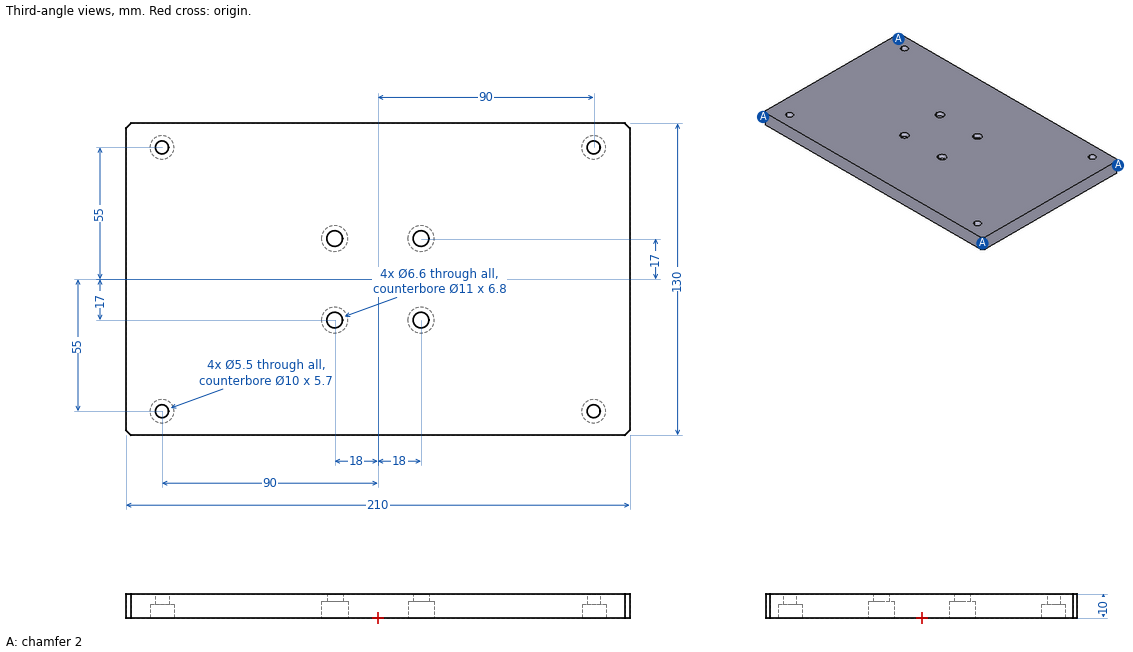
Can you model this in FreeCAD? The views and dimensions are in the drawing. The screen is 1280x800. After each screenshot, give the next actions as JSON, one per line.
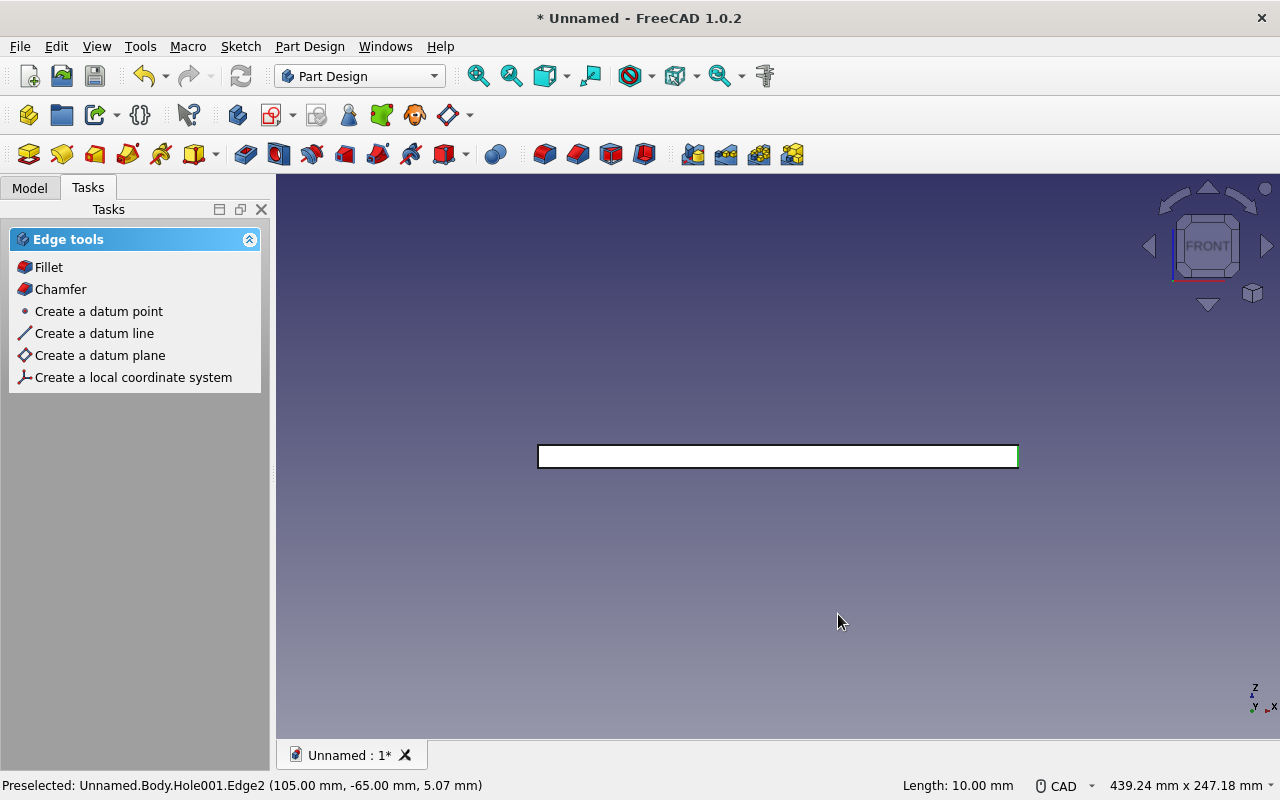
{"action": "left_click", "coordinate": [538, 455], "text": "ctrl"}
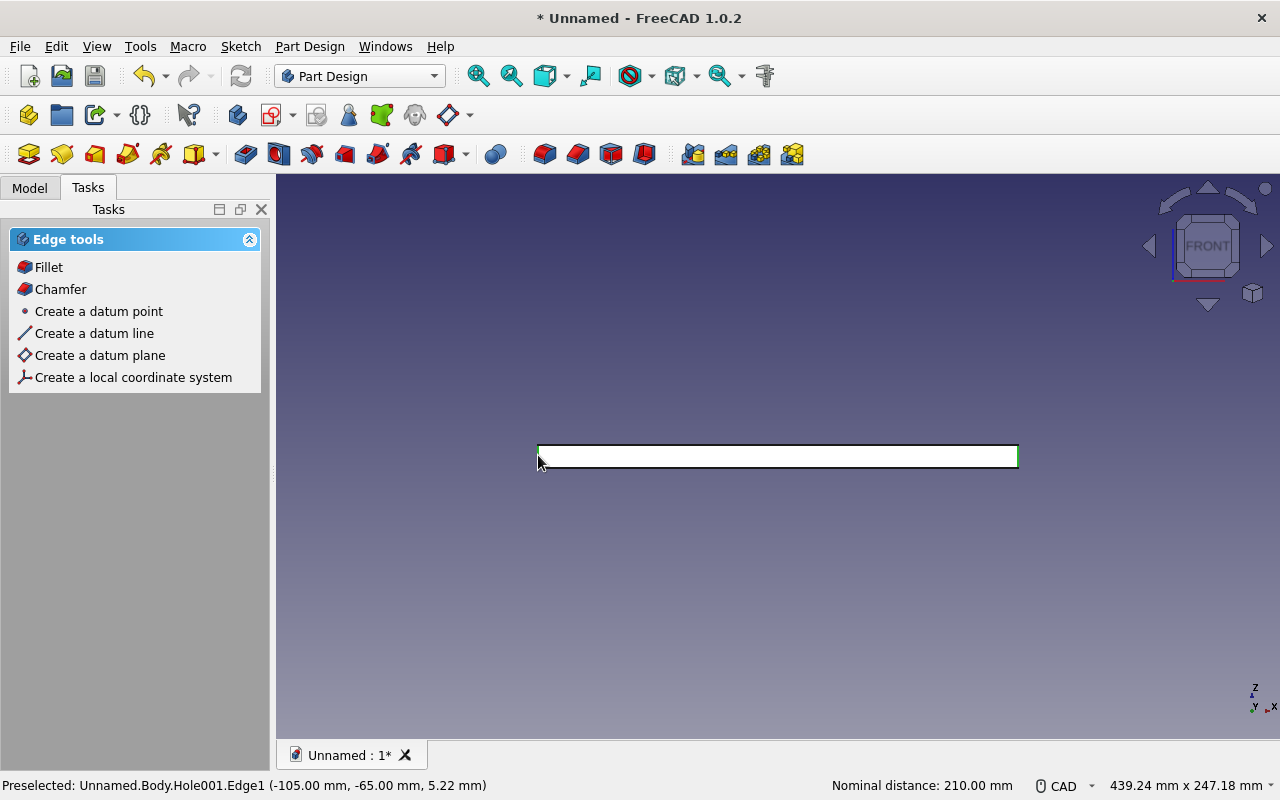
{"action": "key", "text": "3"}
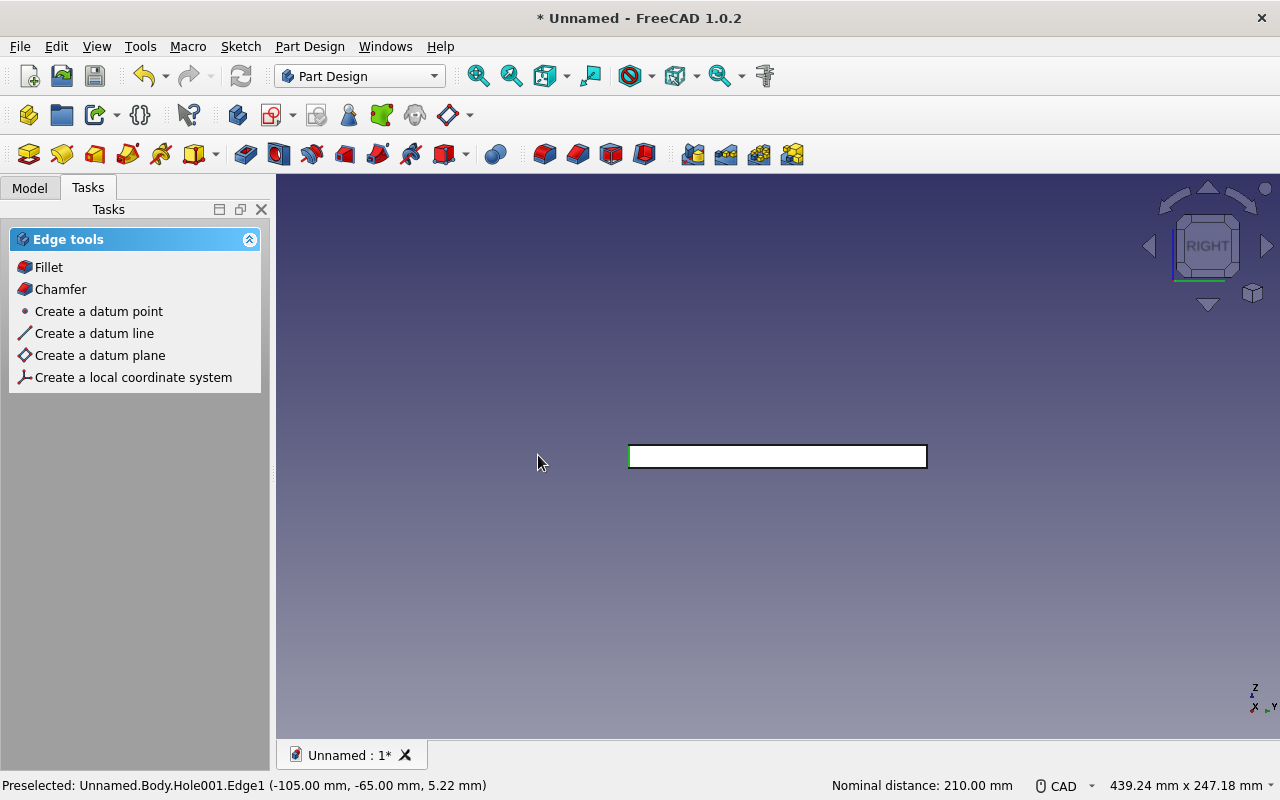
{"action": "left_click", "coordinate": [479, 76]}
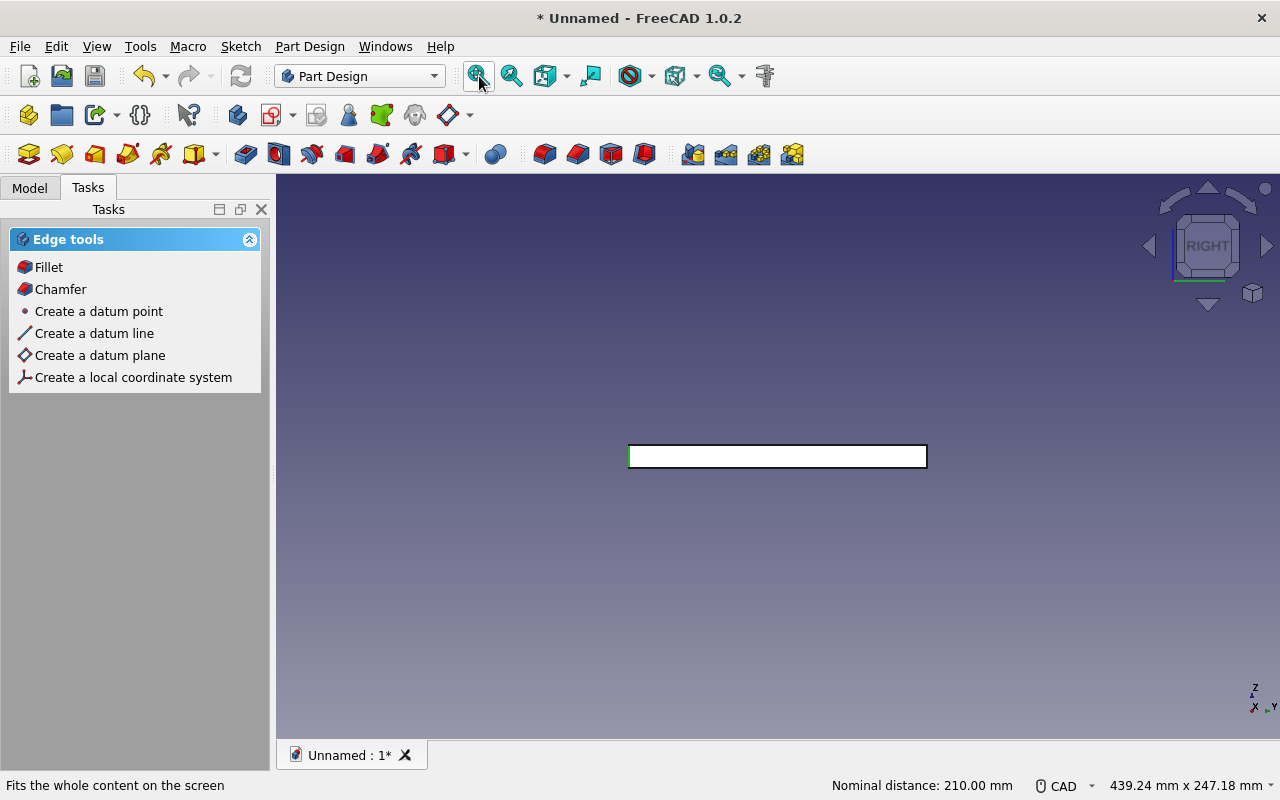
{"action": "left_click", "coordinate": [927, 455], "text": "ctrl"}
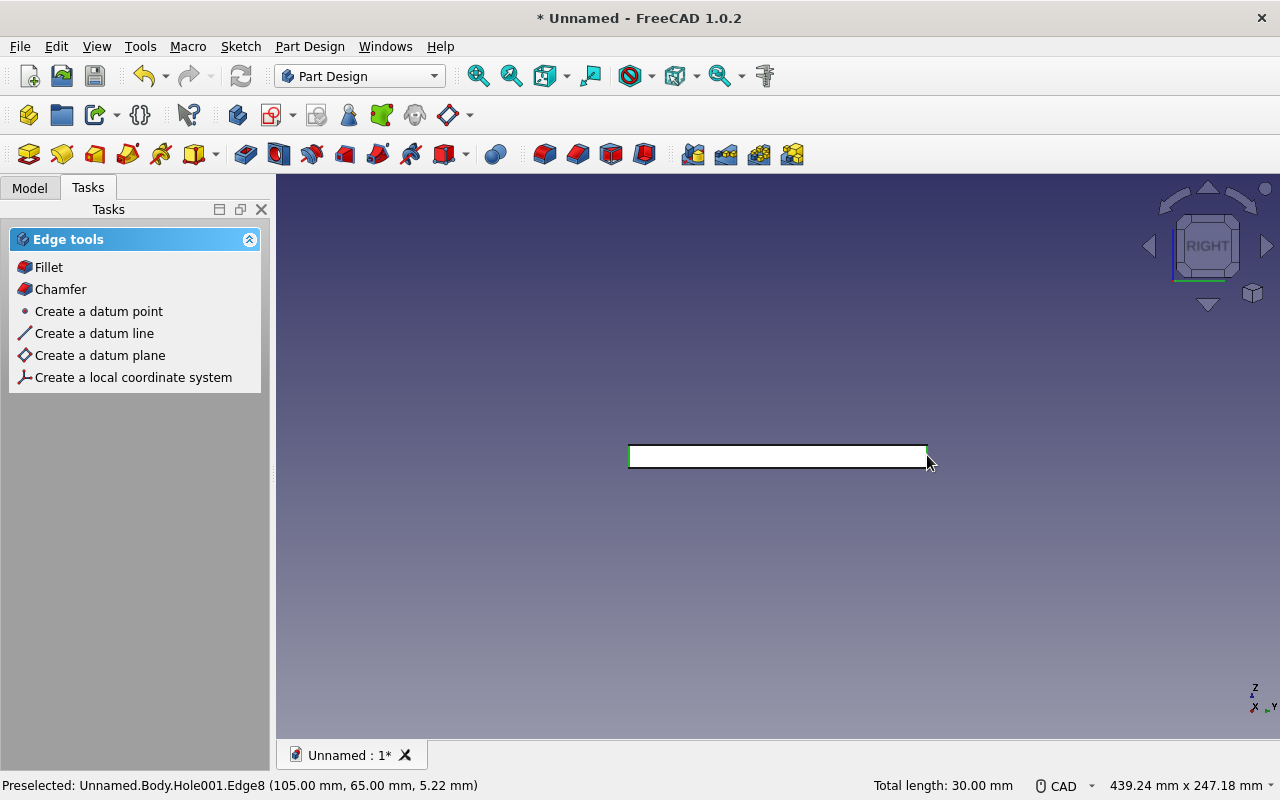
{"action": "key", "text": "5"}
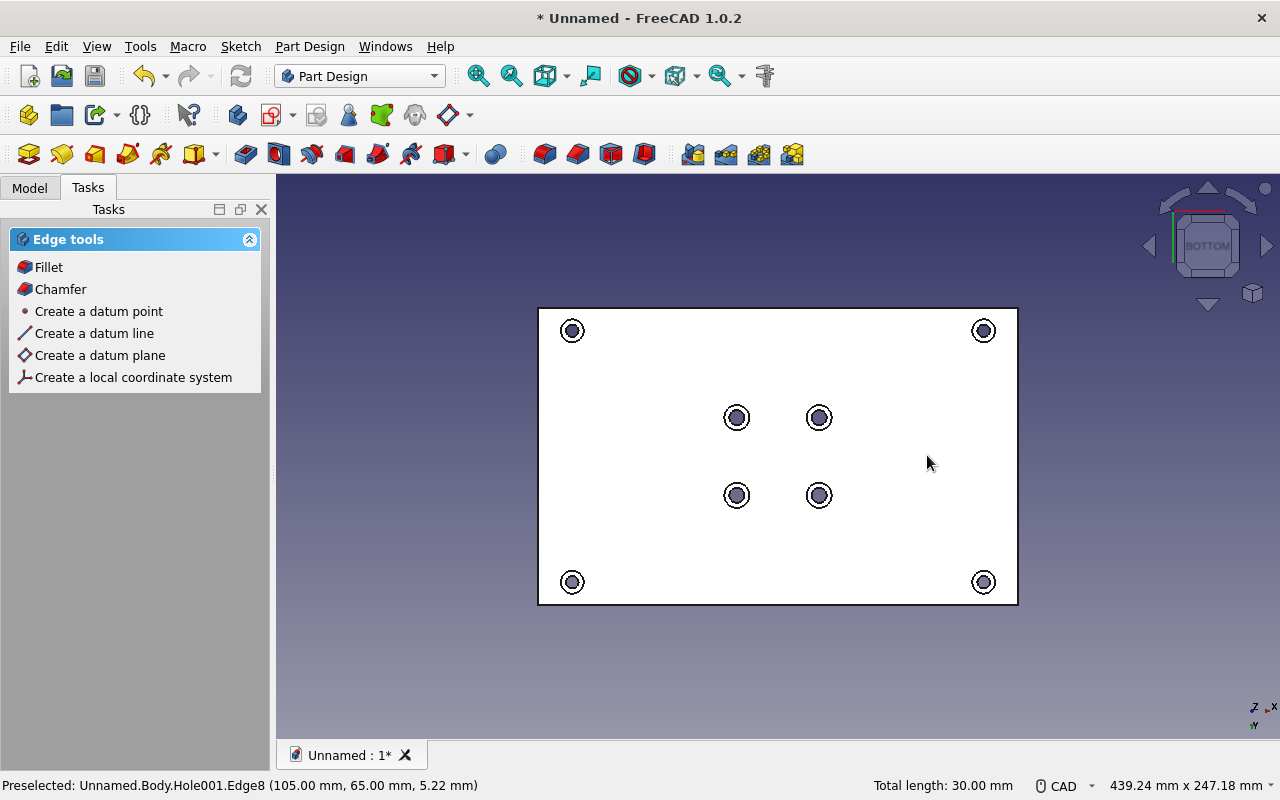
{"action": "key", "text": "4"}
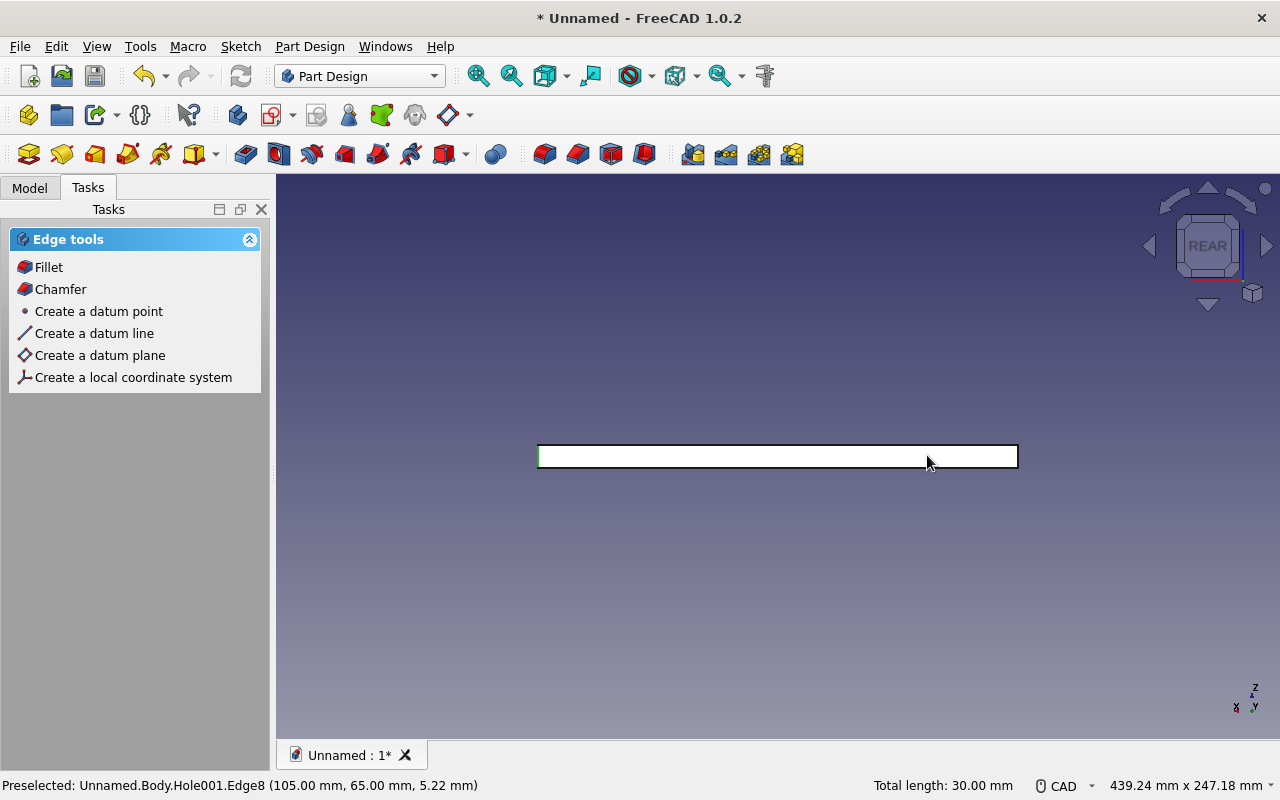
{"action": "left_click", "coordinate": [1018, 455], "text": "ctrl"}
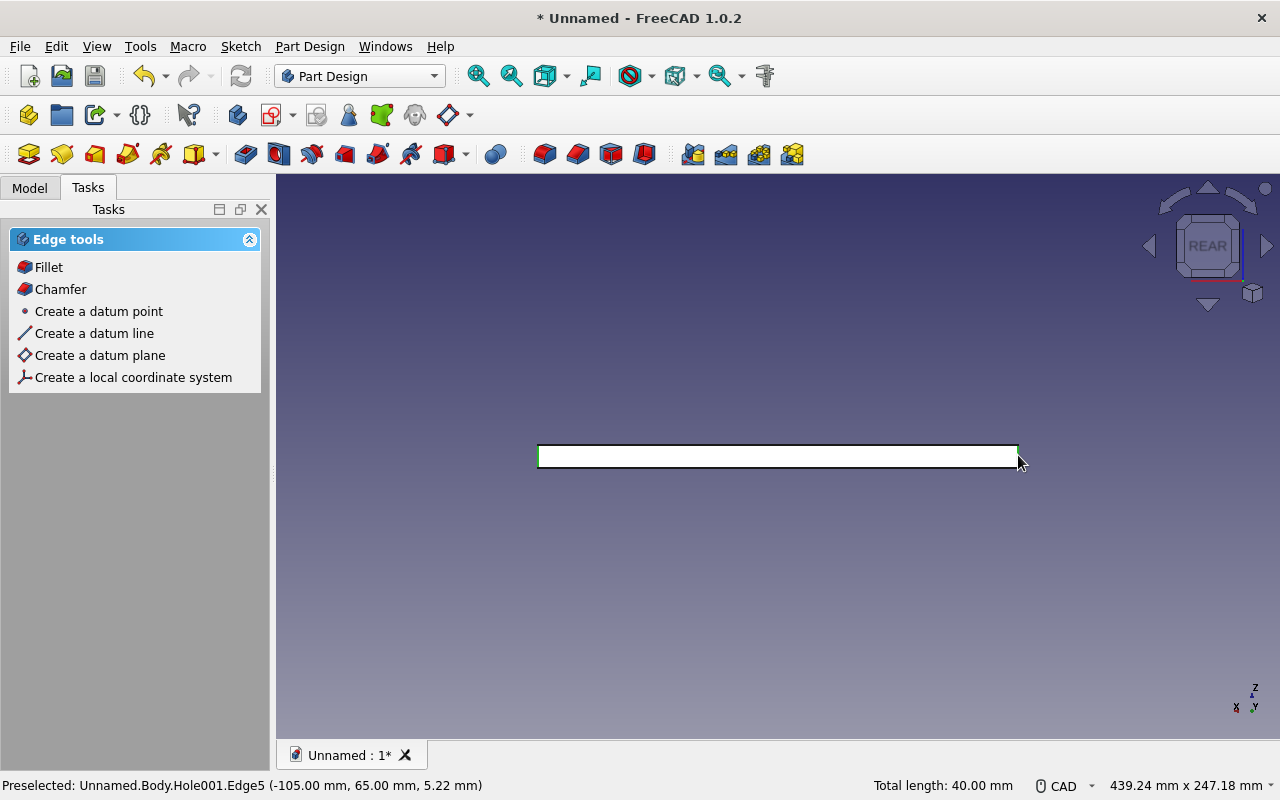
{"action": "left_click", "coordinate": [578, 154]}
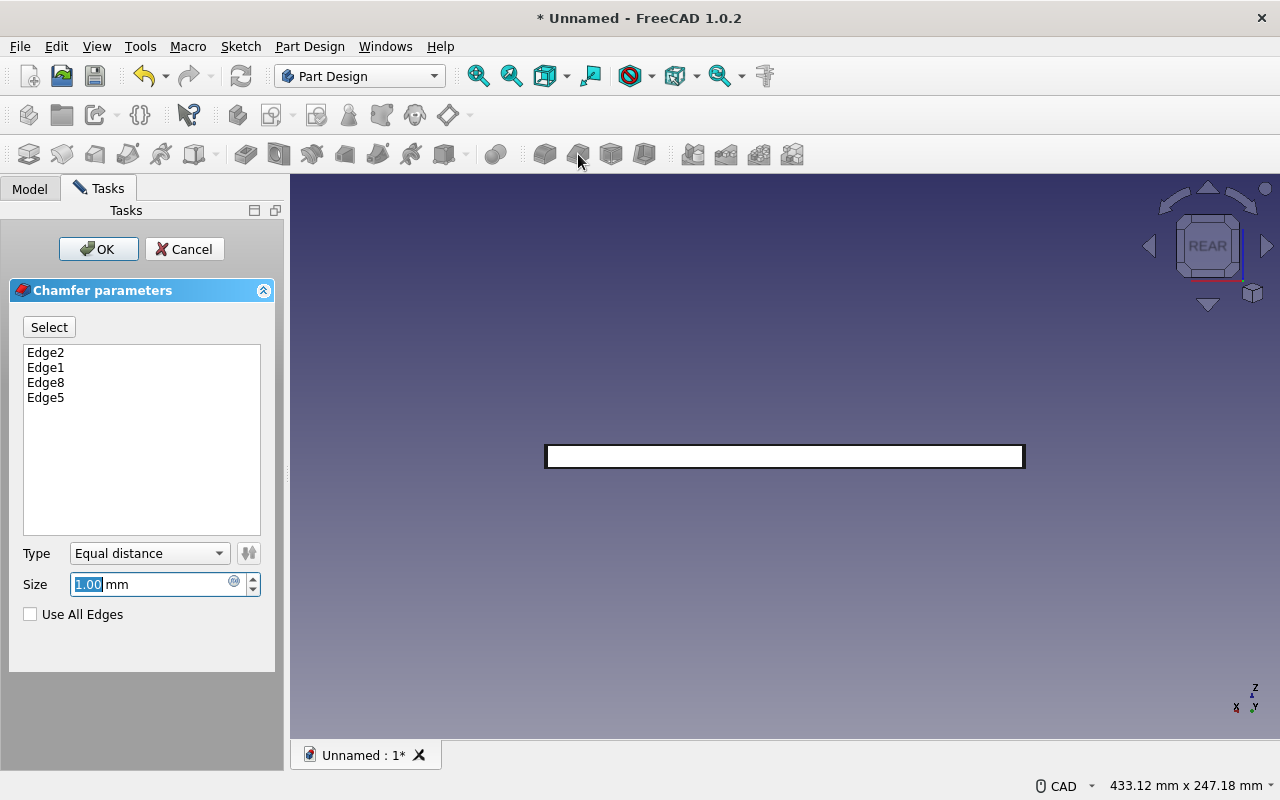
{"action": "type", "text": "2"}
{"action": "key", "text": "Tab"}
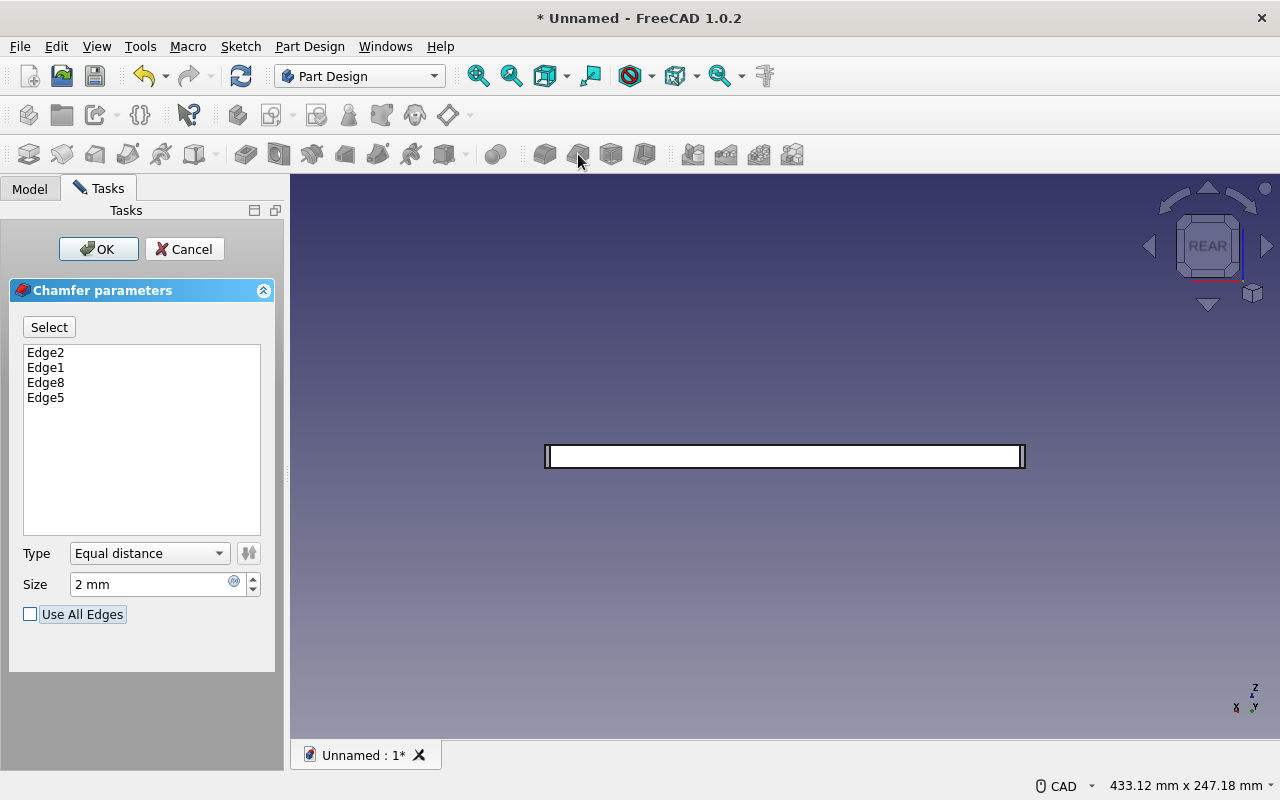
{"action": "left_click", "coordinate": [99, 249]}